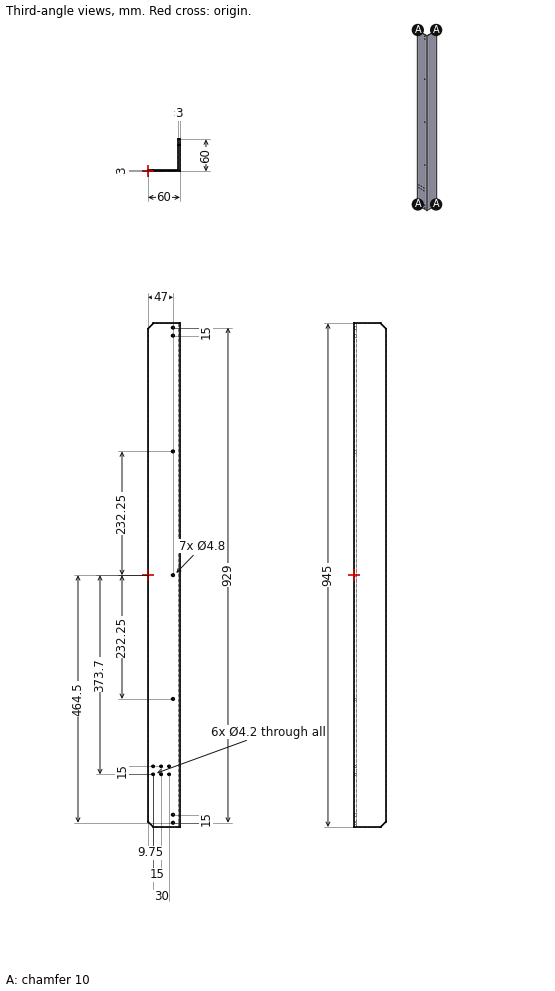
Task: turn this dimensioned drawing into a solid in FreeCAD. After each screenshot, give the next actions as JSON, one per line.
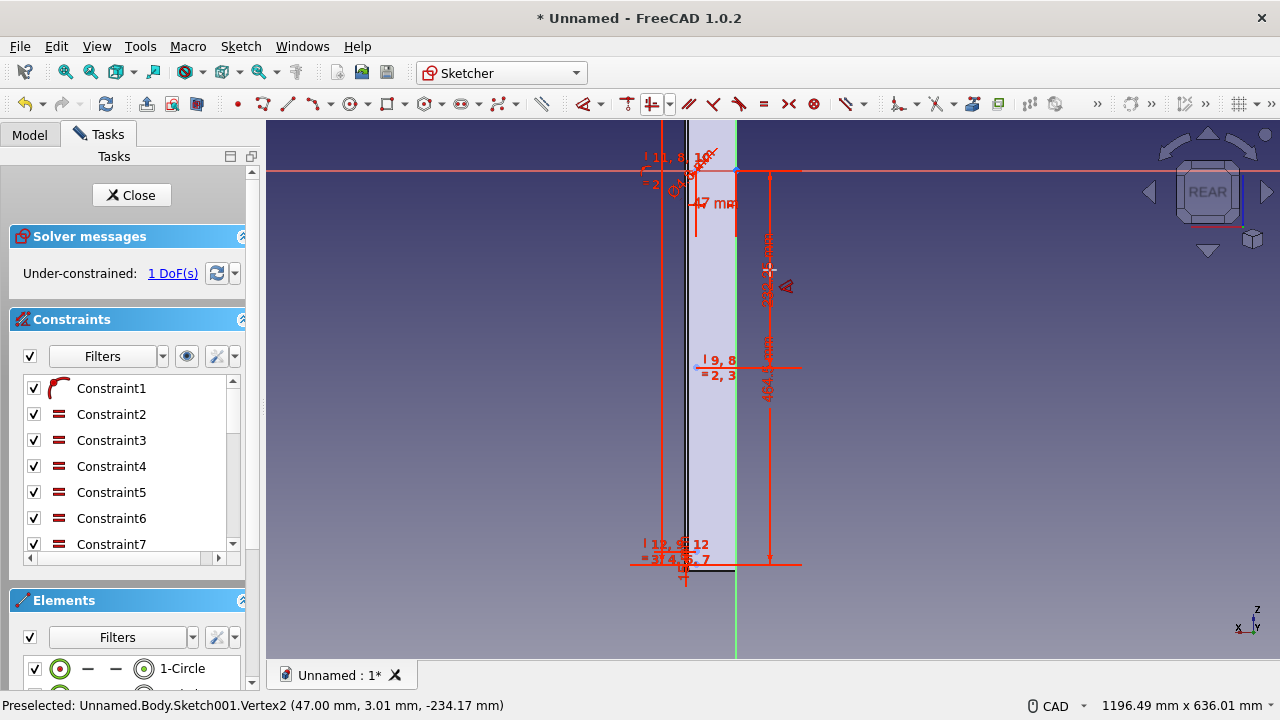
{"action": "scroll", "coordinate": [696, 568], "scroll_direction": "down", "scroll_amount": 4}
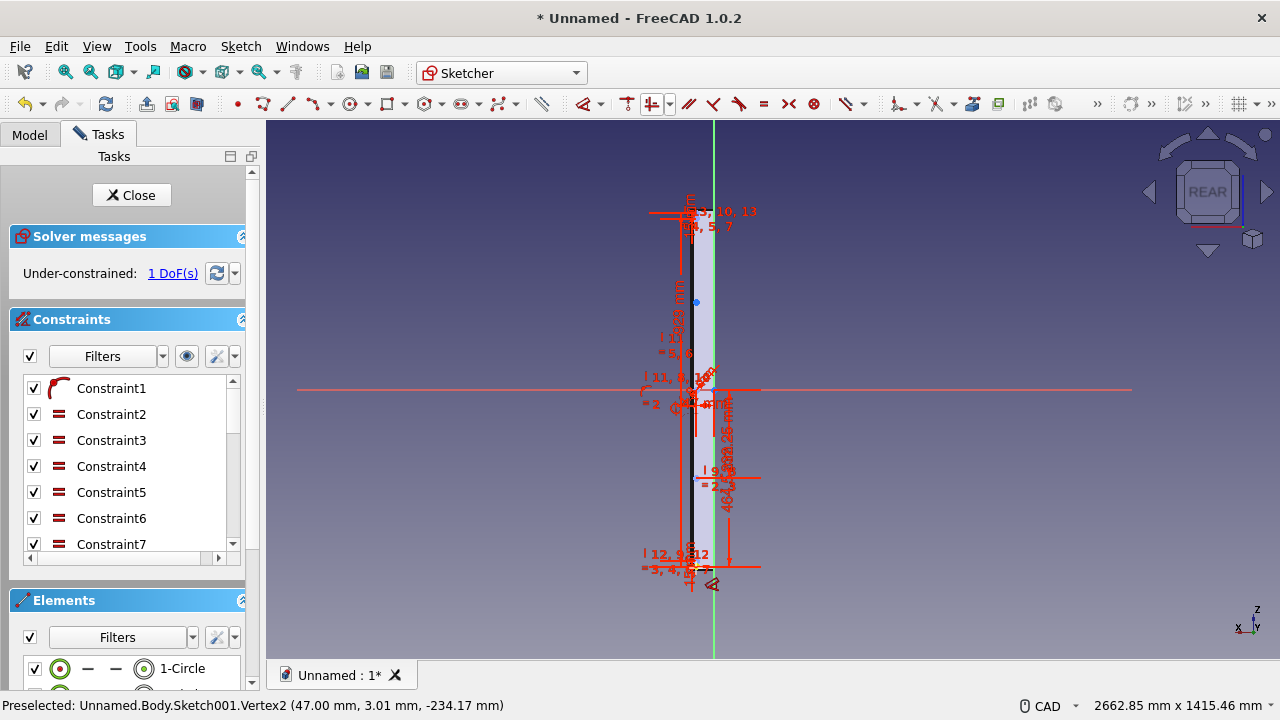
{"action": "left_click", "coordinate": [696, 302]}
{"action": "left_click", "coordinate": [748, 346]}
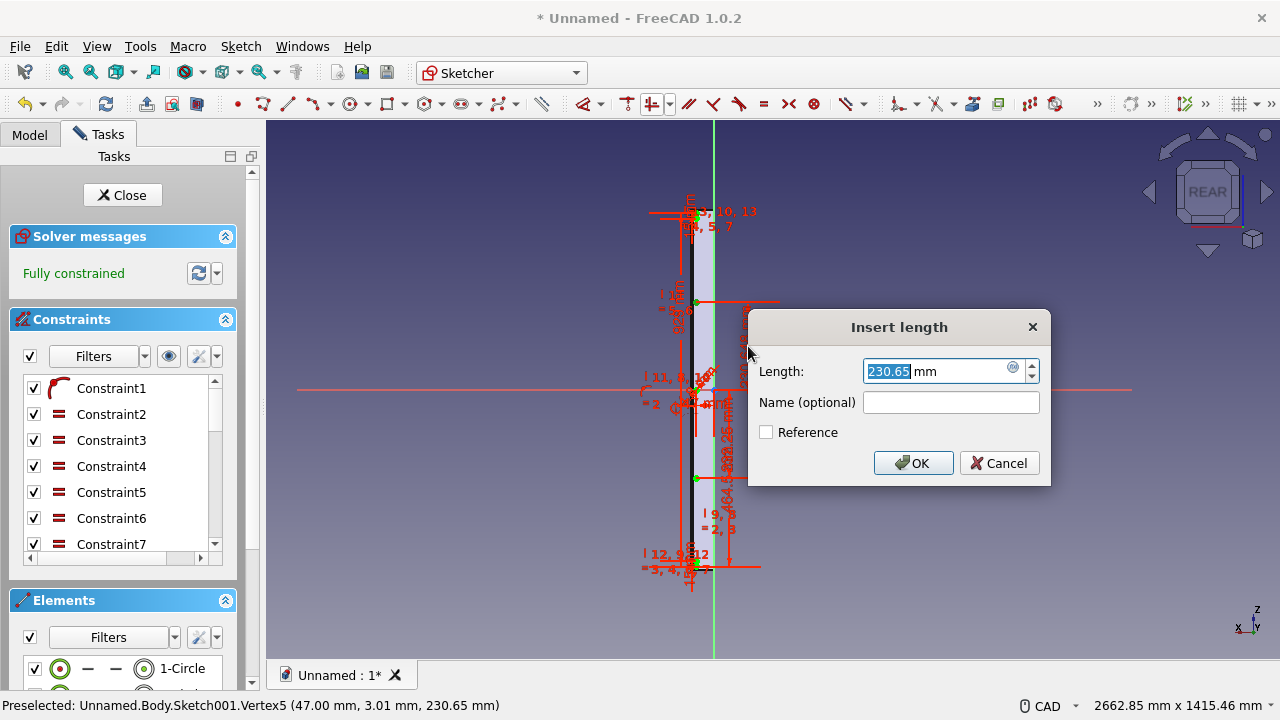
{"action": "type", "text": "232.25"}
{"action": "key", "text": "Return"}
{"action": "key", "text": "Escape"}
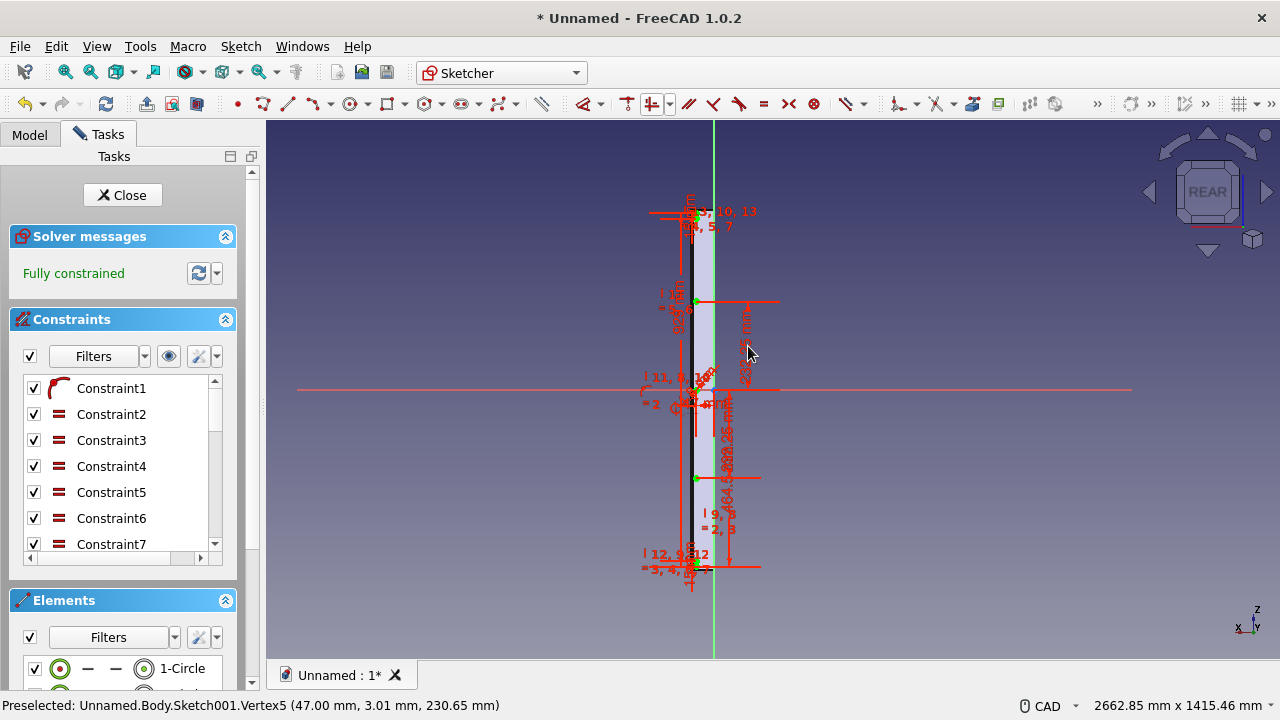
{"action": "left_click", "coordinate": [123, 195]}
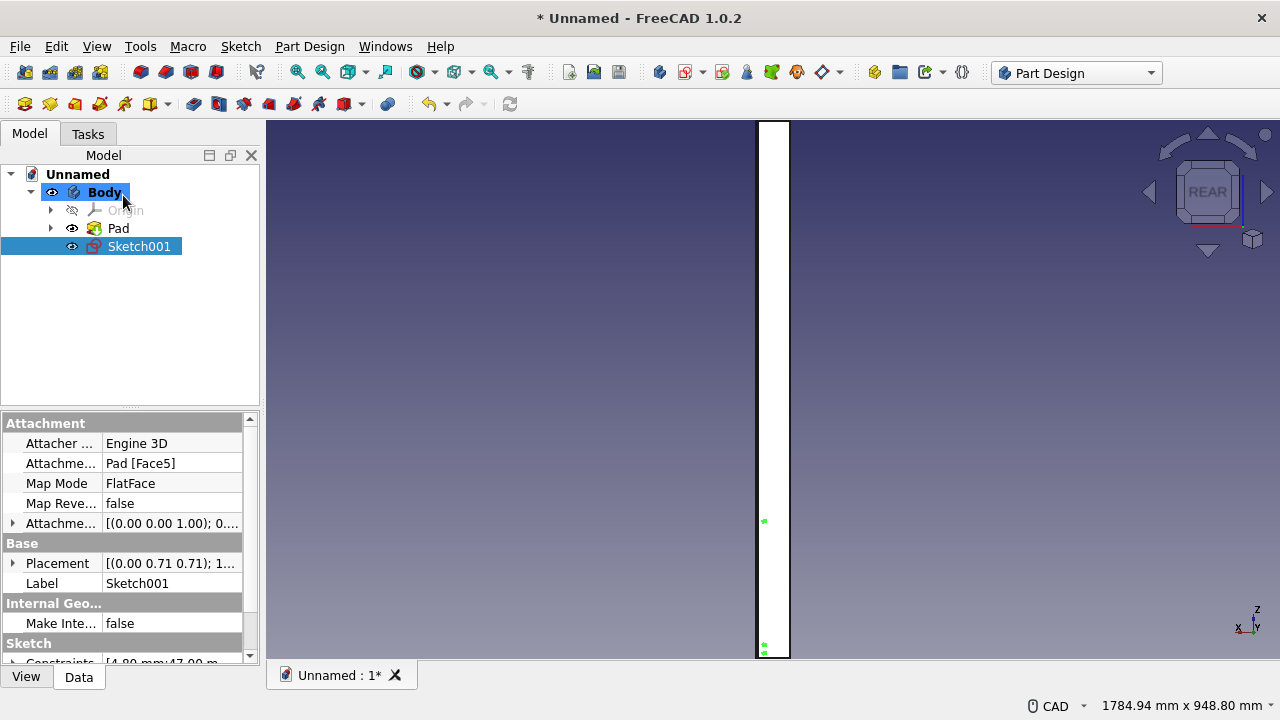
{"action": "left_click", "coordinate": [194, 104]}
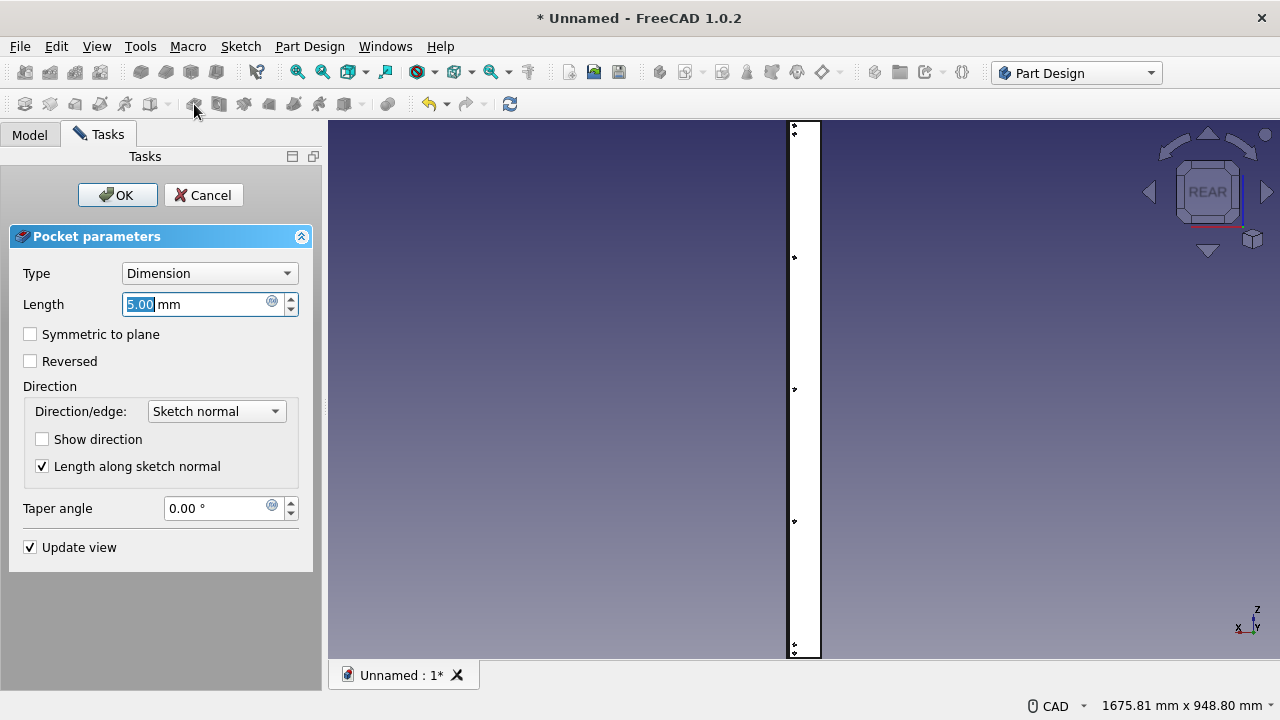
{"action": "left_click", "coordinate": [210, 274]}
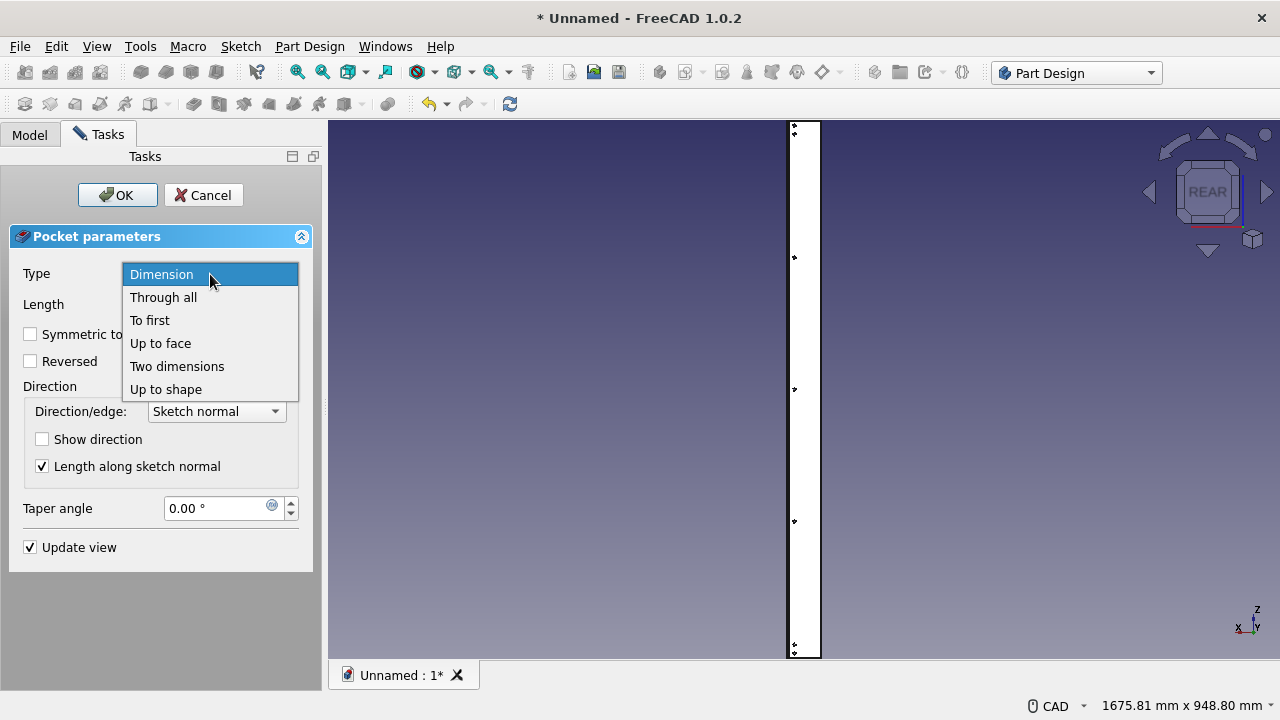
{"action": "left_click", "coordinate": [208, 298]}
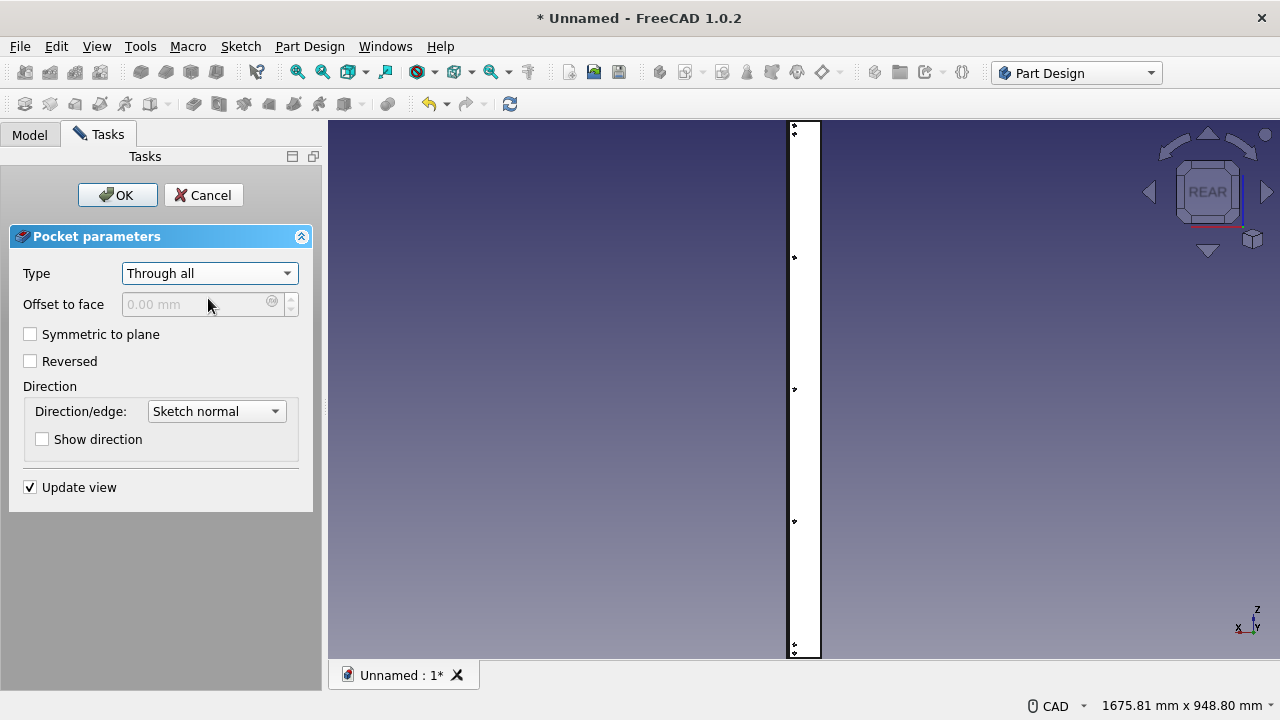
{"action": "left_click", "coordinate": [118, 195]}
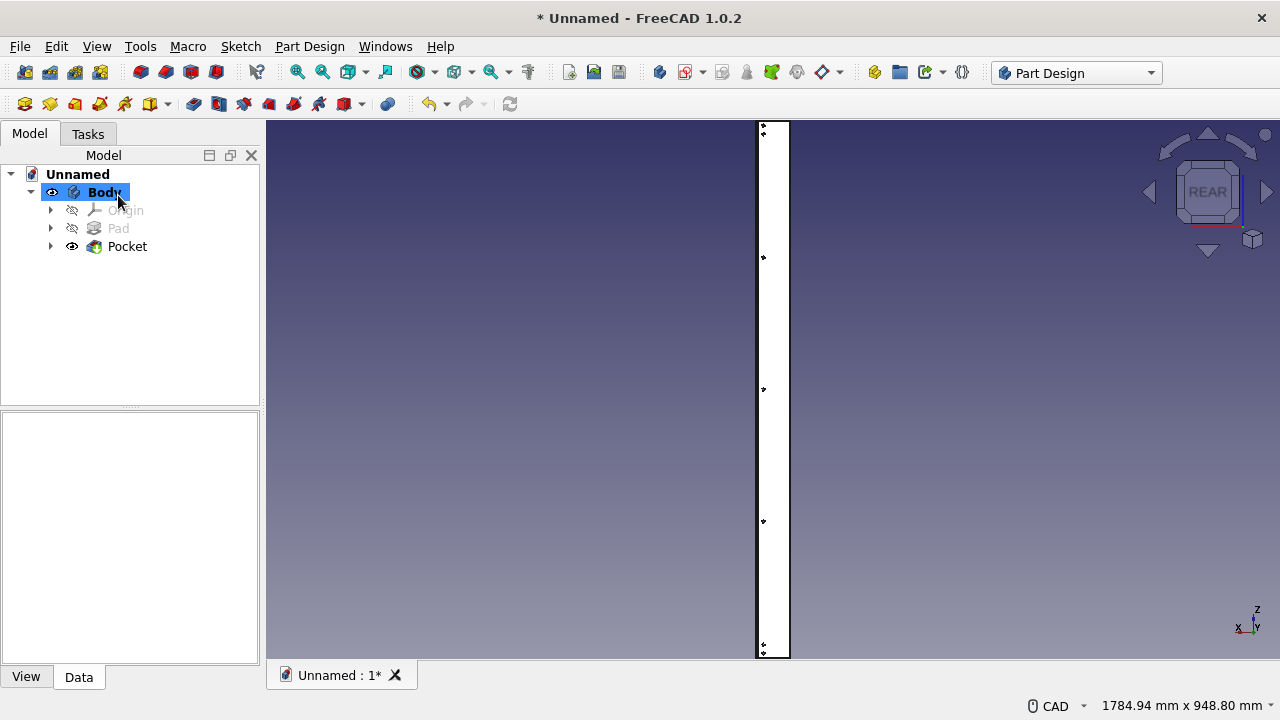
{"action": "key", "text": "0"}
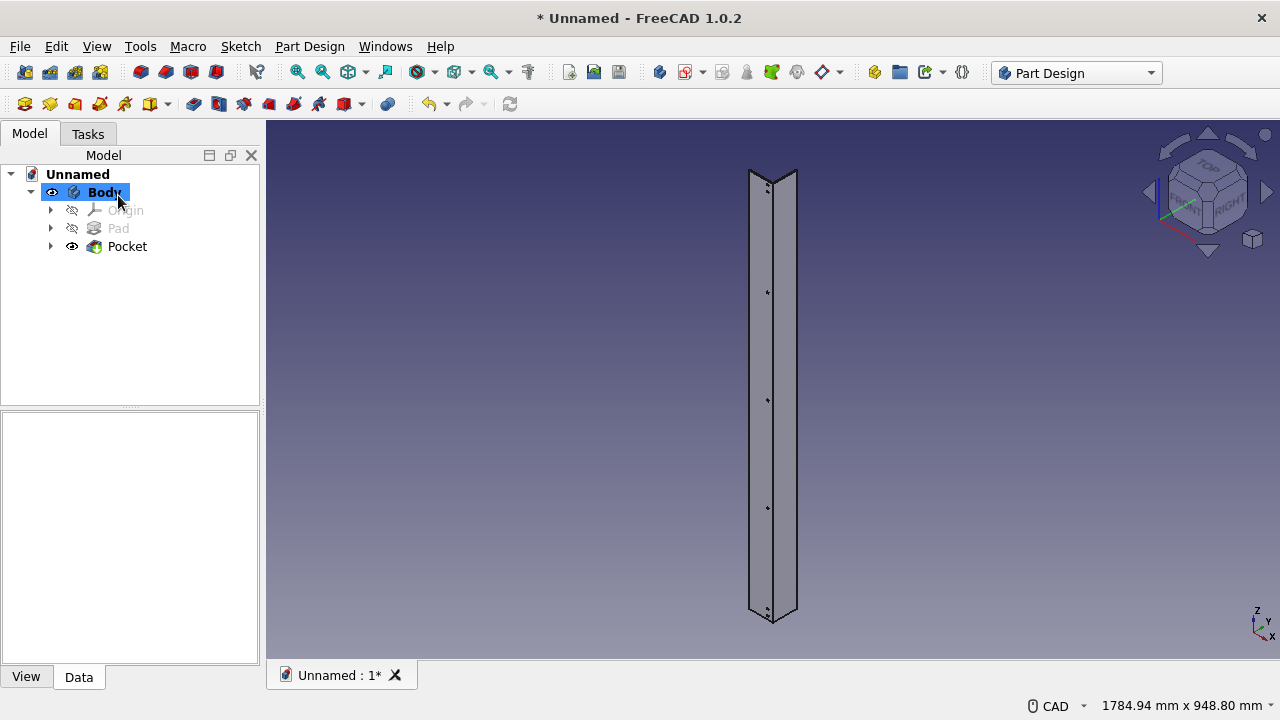
{"action": "scroll", "coordinate": [796, 169], "scroll_direction": "up", "scroll_amount": 15}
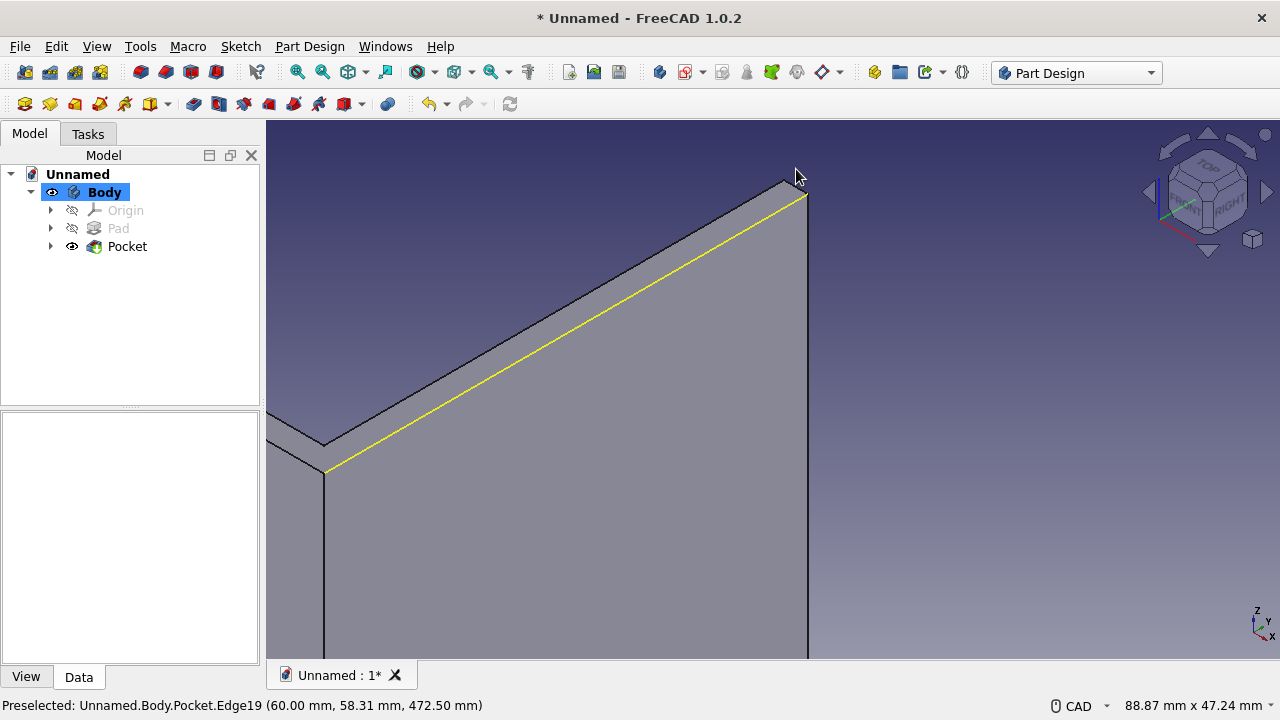
{"action": "left_click", "coordinate": [298, 72]}